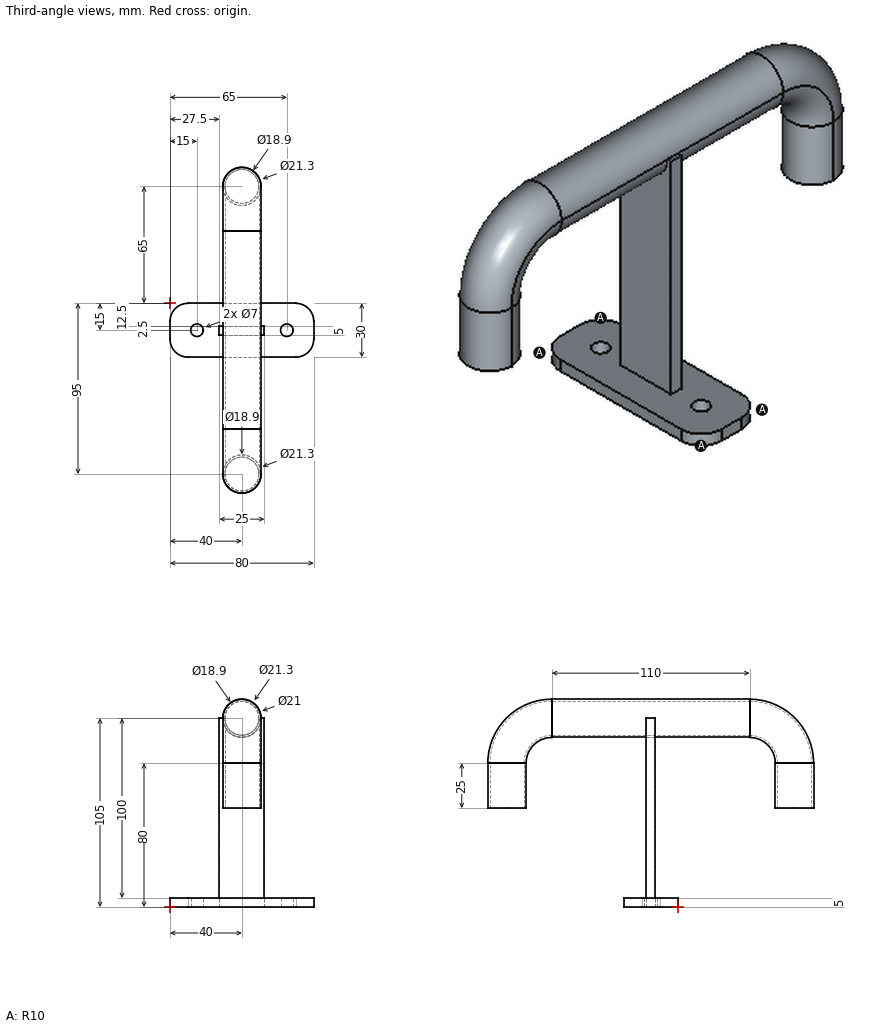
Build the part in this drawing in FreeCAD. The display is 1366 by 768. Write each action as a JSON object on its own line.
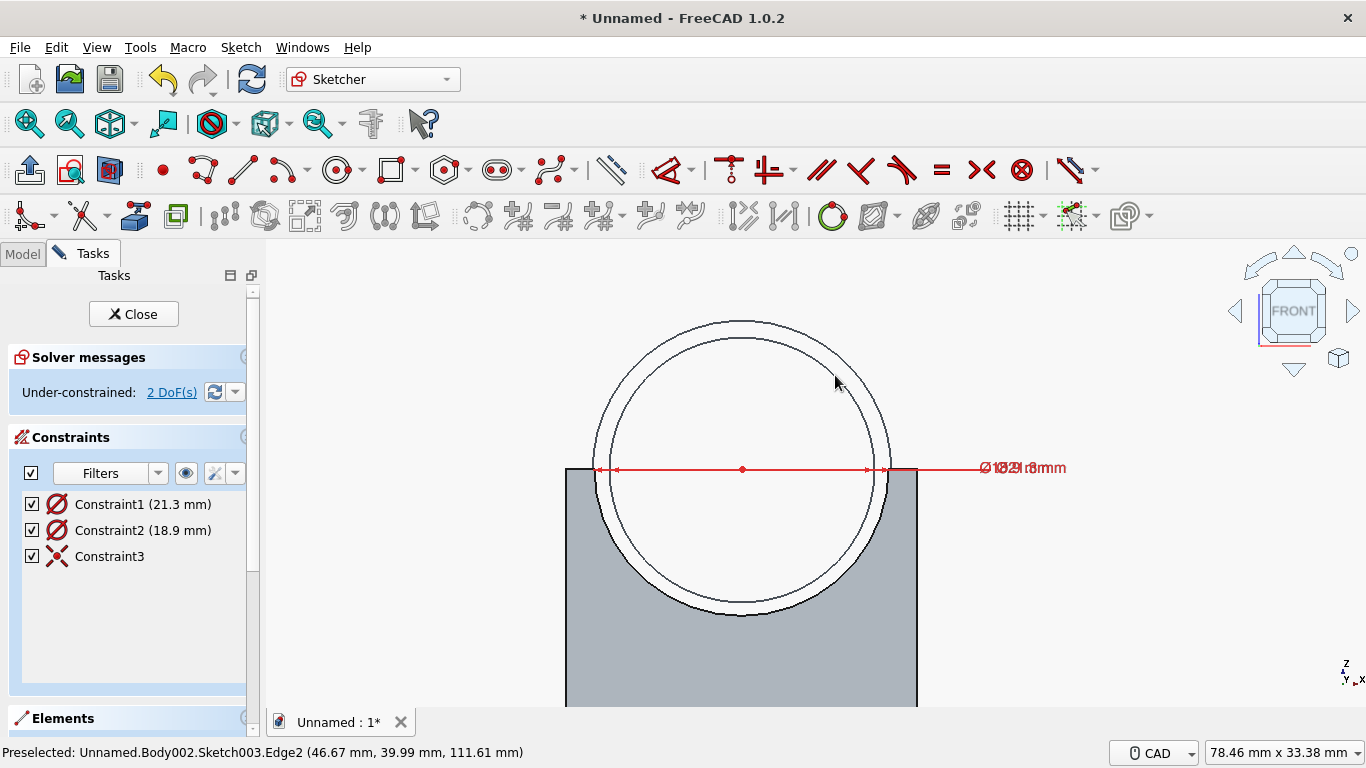
{"action": "left_click", "coordinate": [666, 170]}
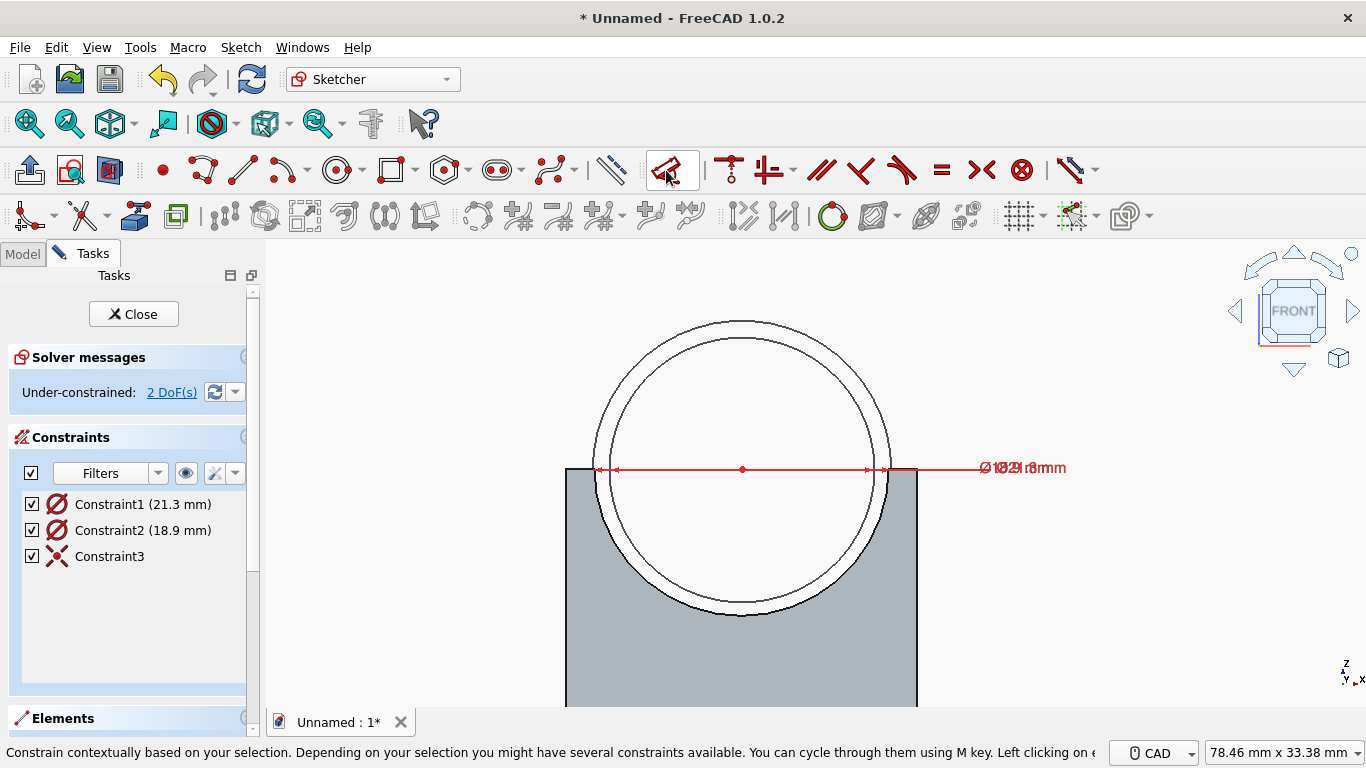
{"action": "left_click", "coordinate": [742, 470]}
{"action": "left_click", "coordinate": [518, 436]}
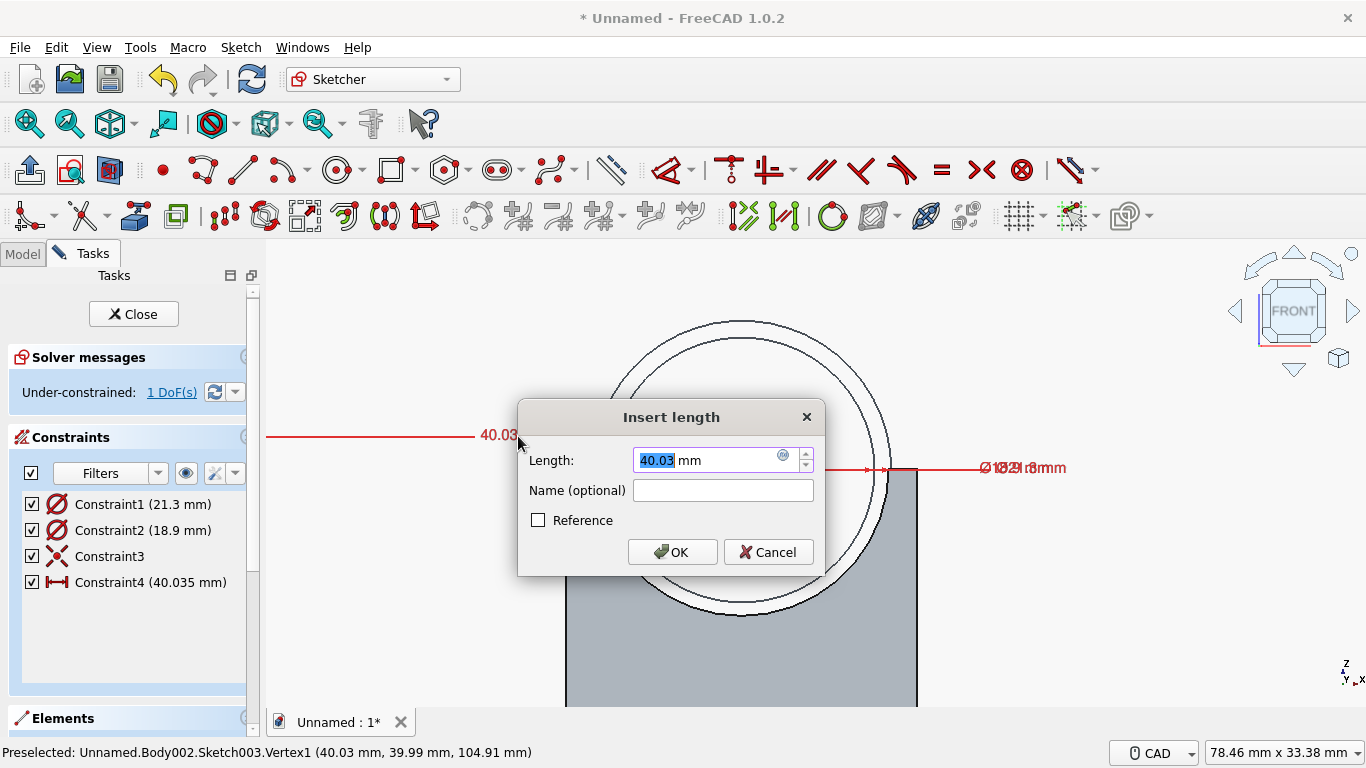
{"action": "type", "text": "40"}
{"action": "key", "text": "Return"}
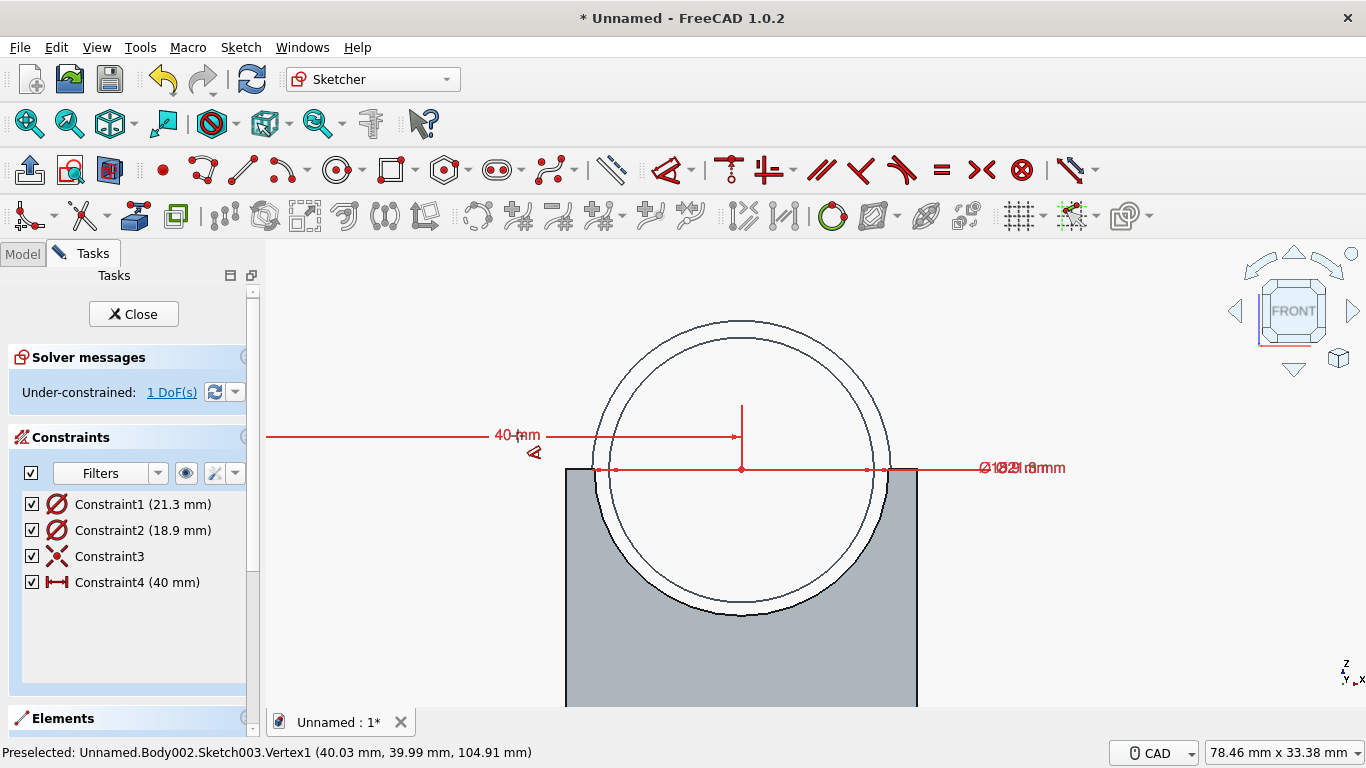
{"action": "left_click", "coordinate": [742, 470]}
{"action": "left_click", "coordinate": [776, 575]}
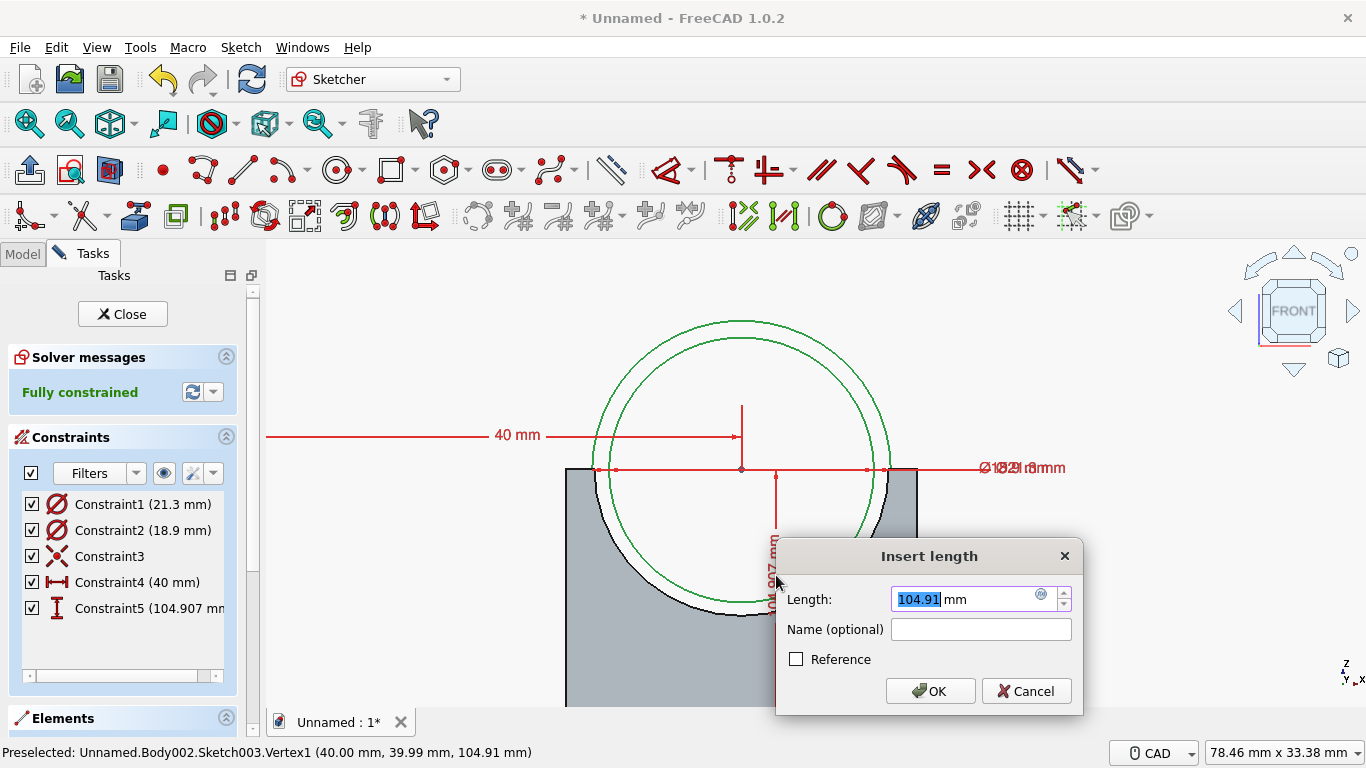
{"action": "type", "text": "105"}
{"action": "key", "text": "Return"}
{"action": "key", "text": "Escape"}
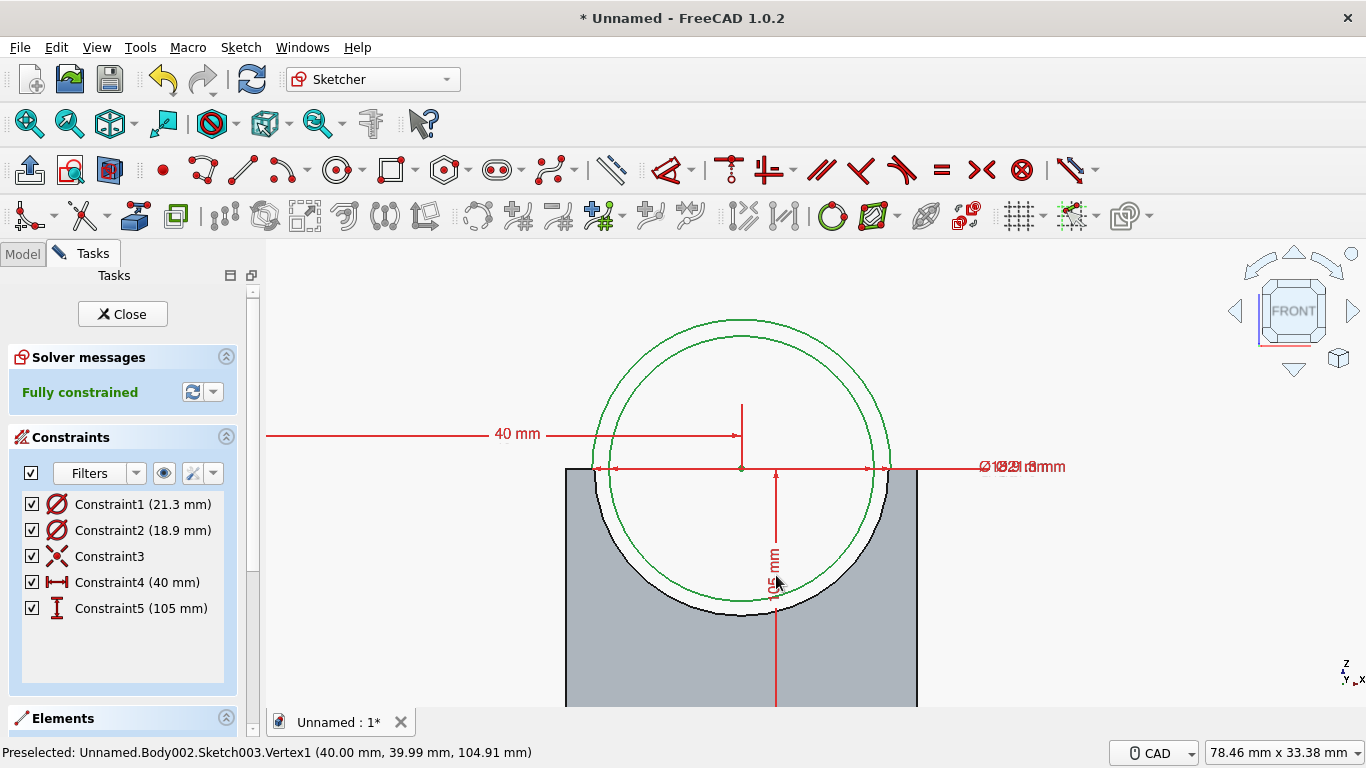
{"action": "left_click", "coordinate": [123, 314]}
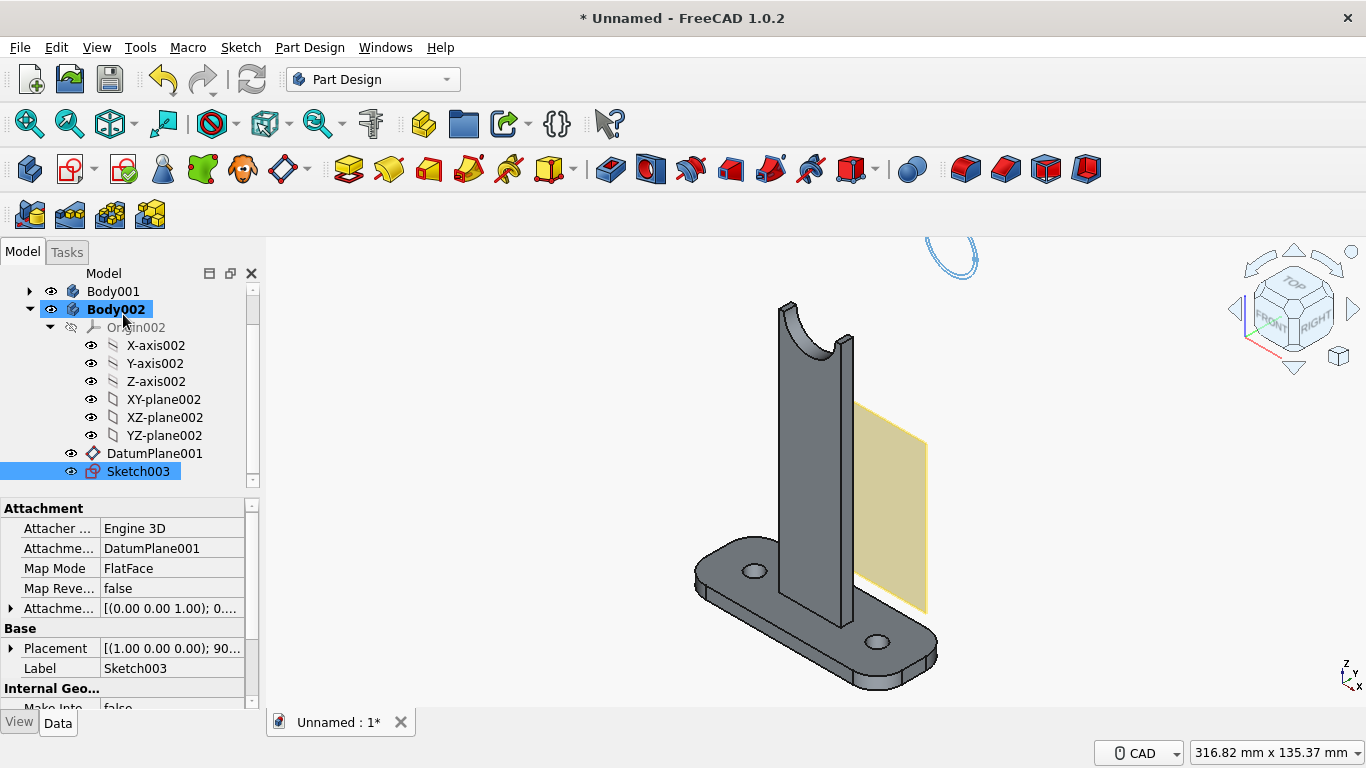
{"action": "left_click", "coordinate": [350, 170]}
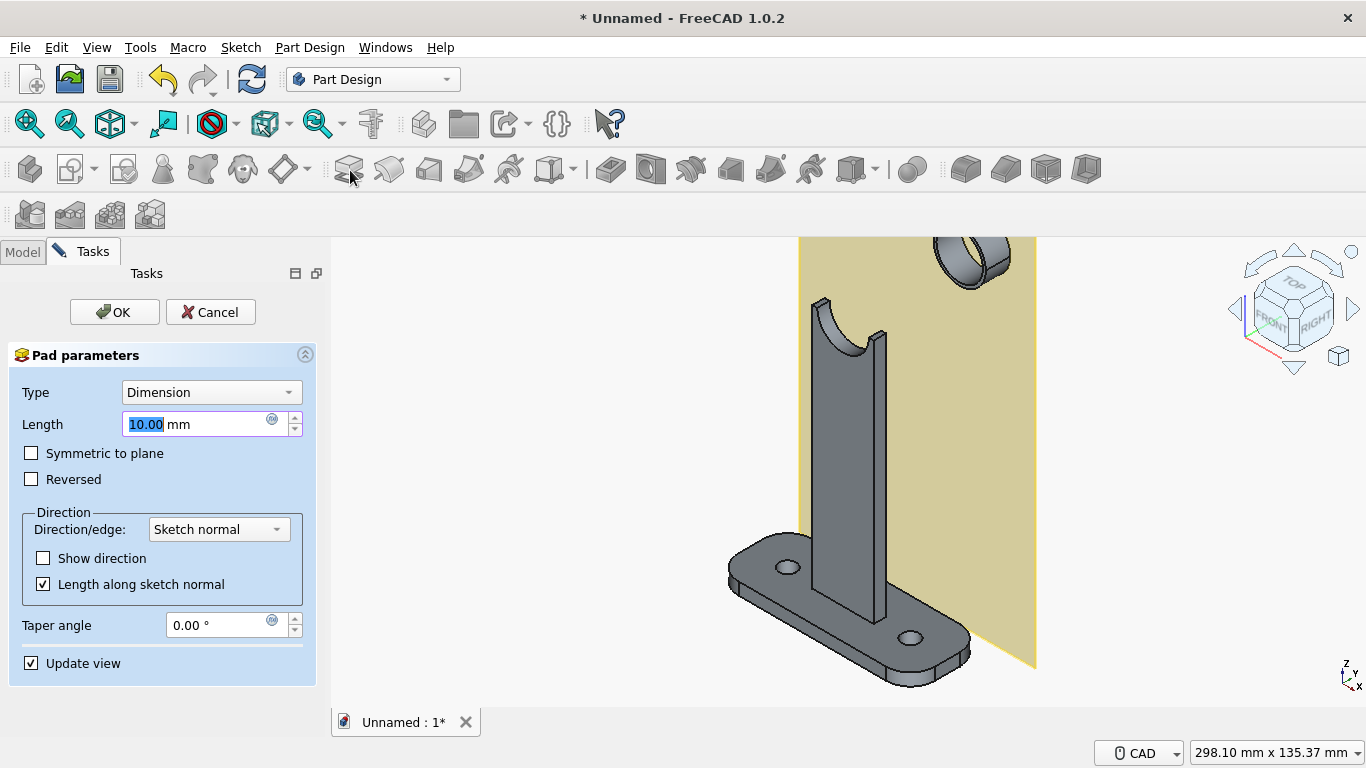
{"action": "type", "text": "110"}
{"action": "key", "text": "Tab"}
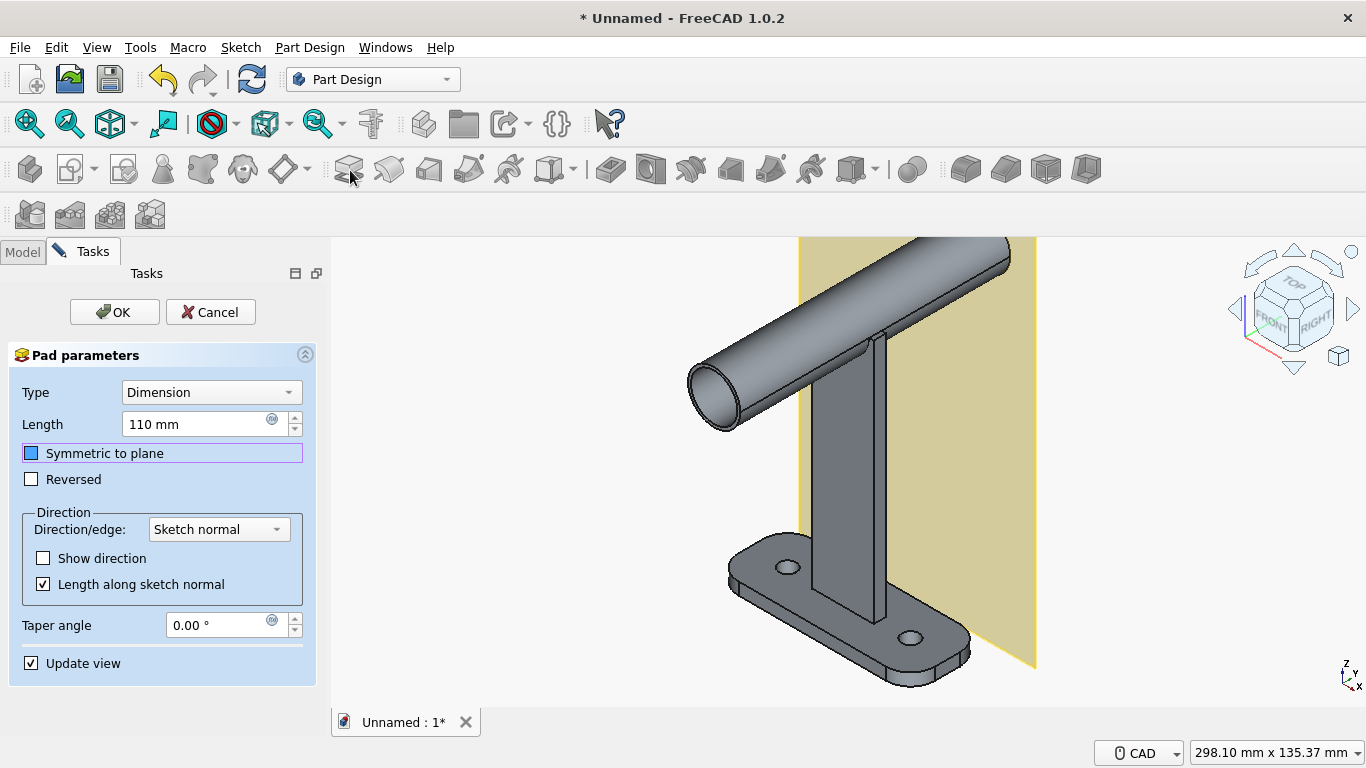
{"action": "left_click", "coordinate": [115, 312]}